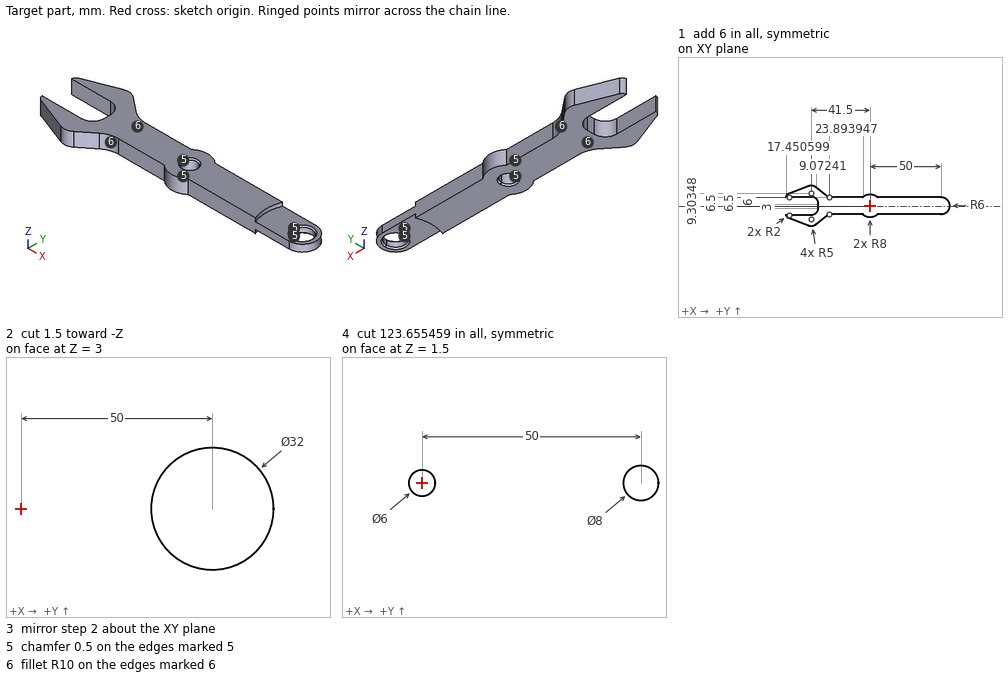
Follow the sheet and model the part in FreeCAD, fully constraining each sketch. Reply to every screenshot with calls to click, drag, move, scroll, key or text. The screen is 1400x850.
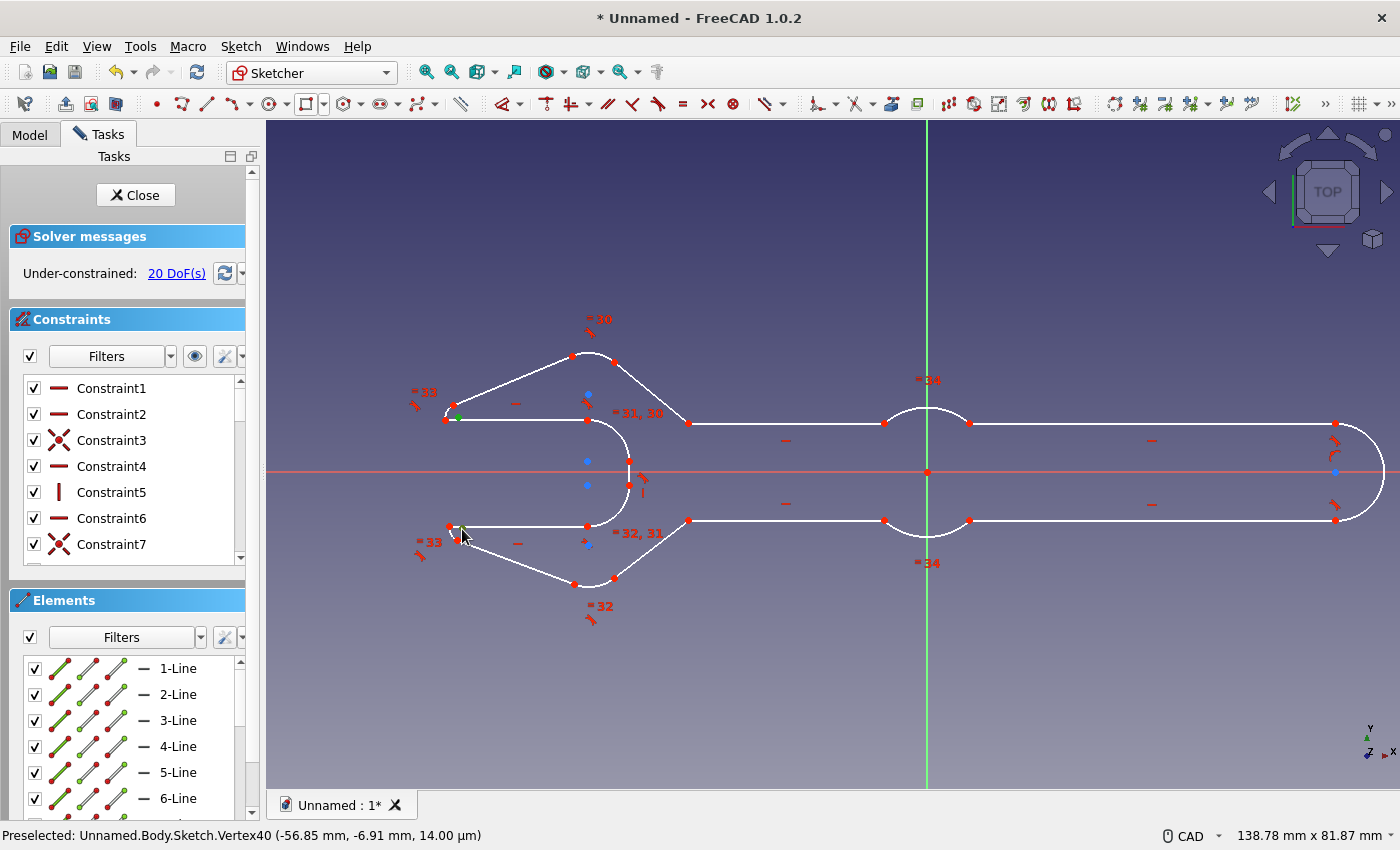
click(361, 472)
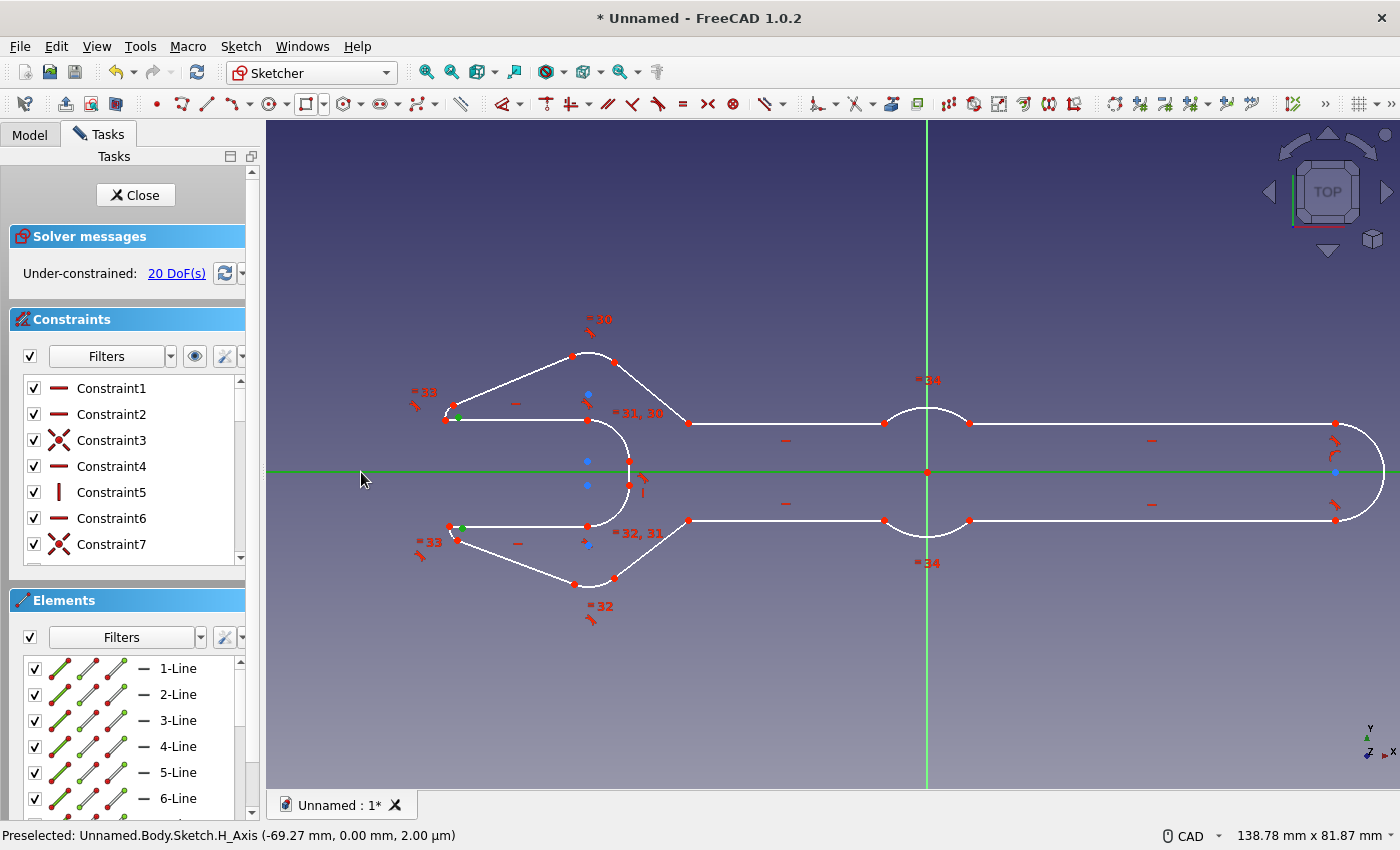
click(708, 104)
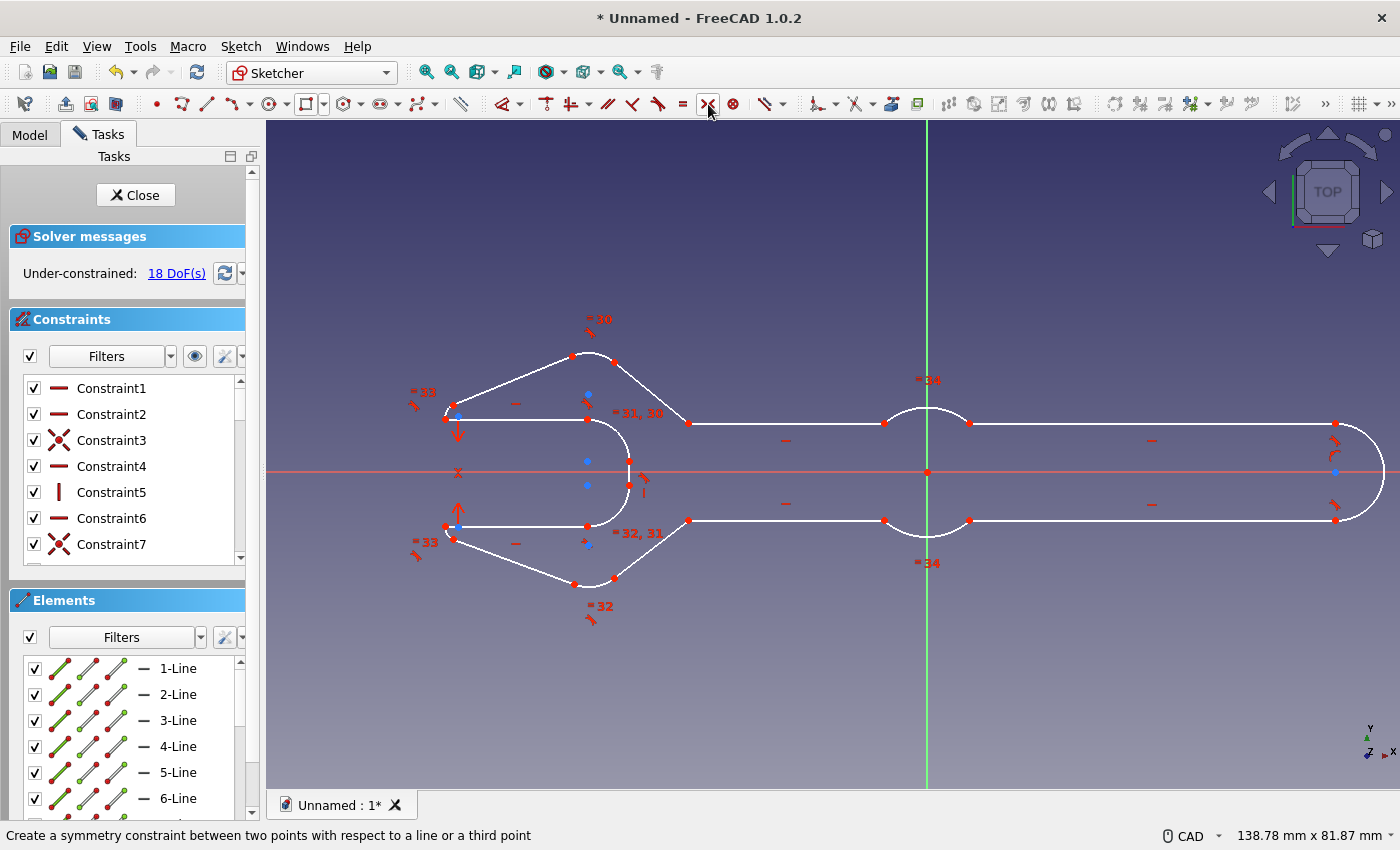
click(588, 394)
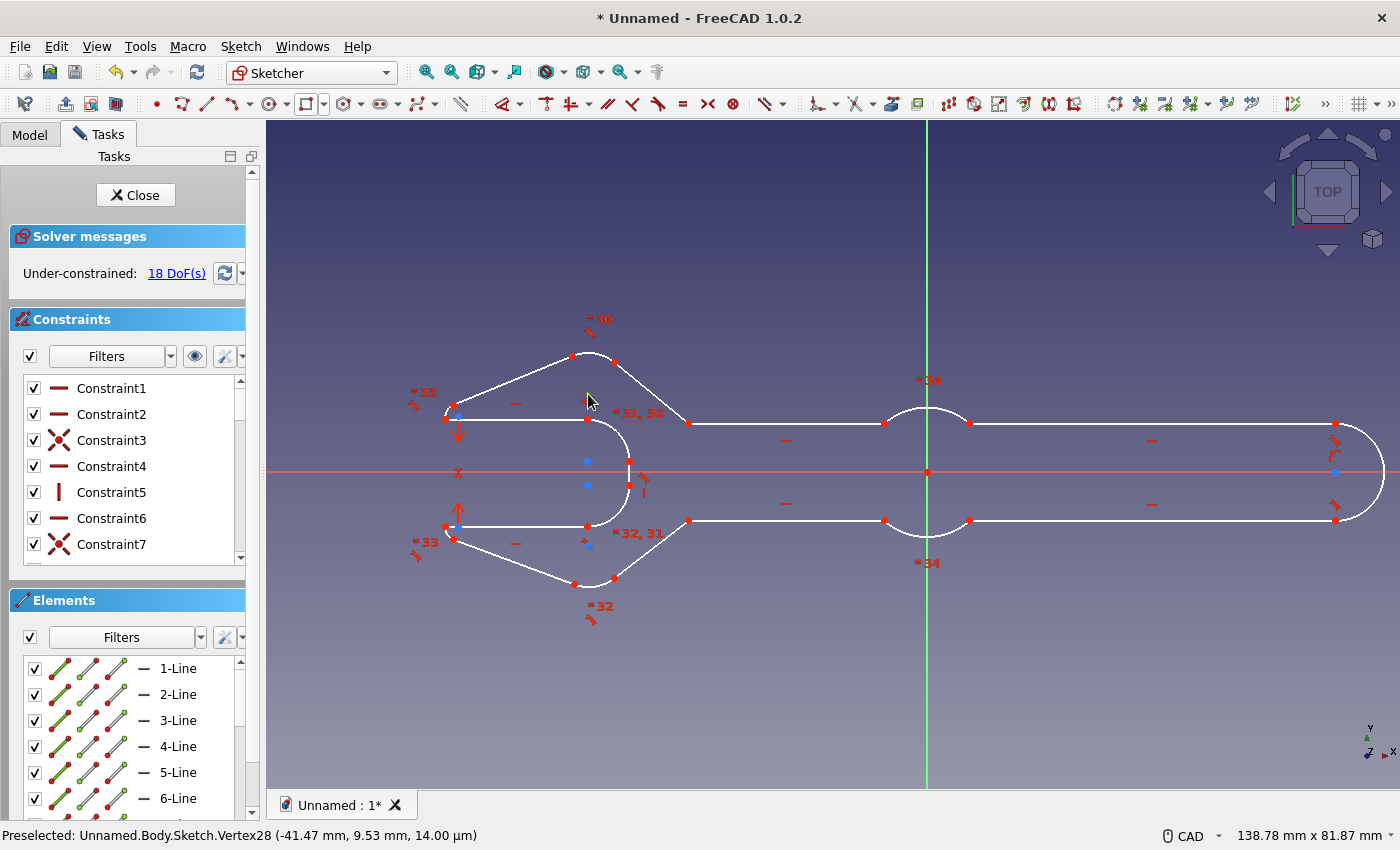
click(589, 546)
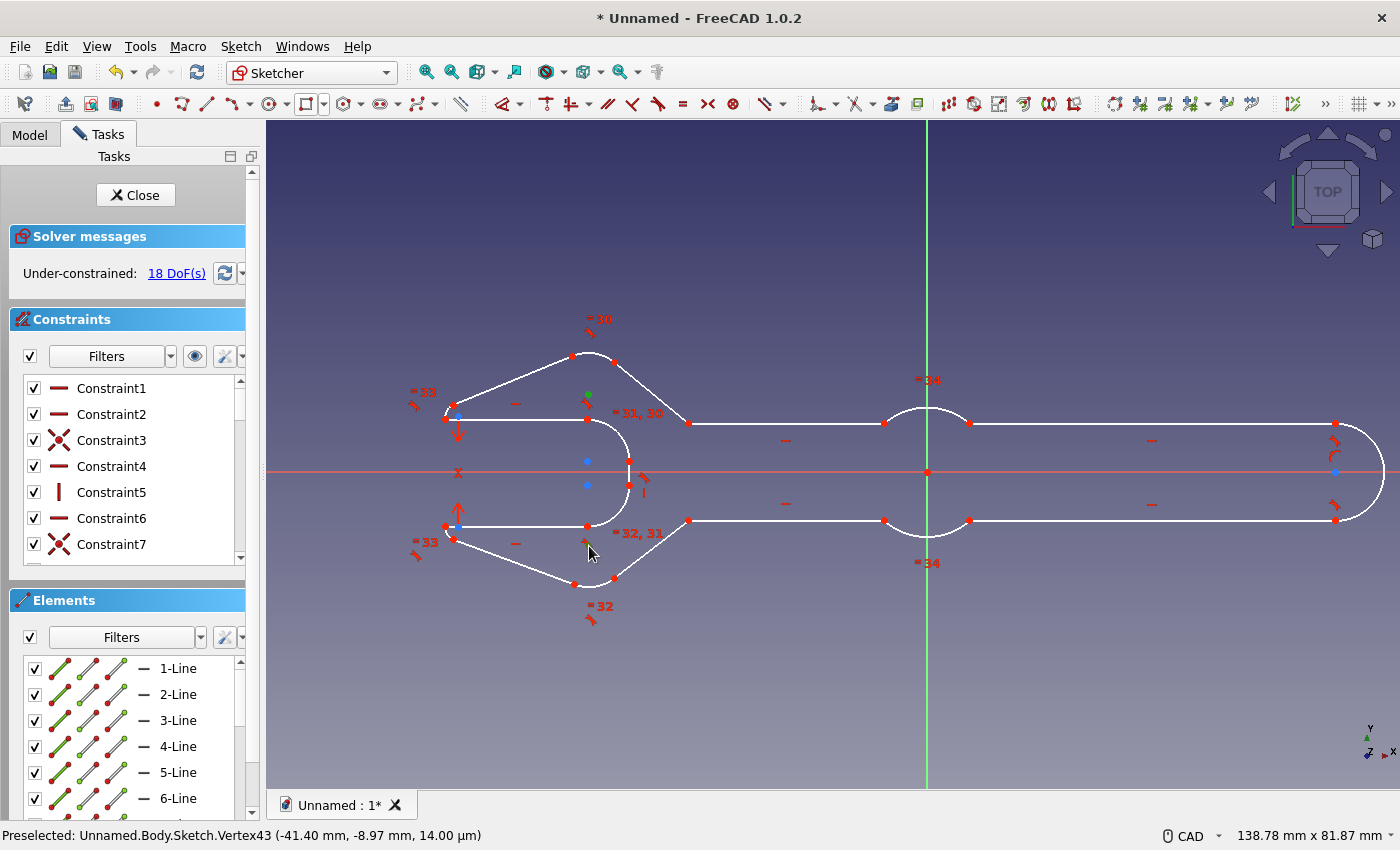
click(361, 472)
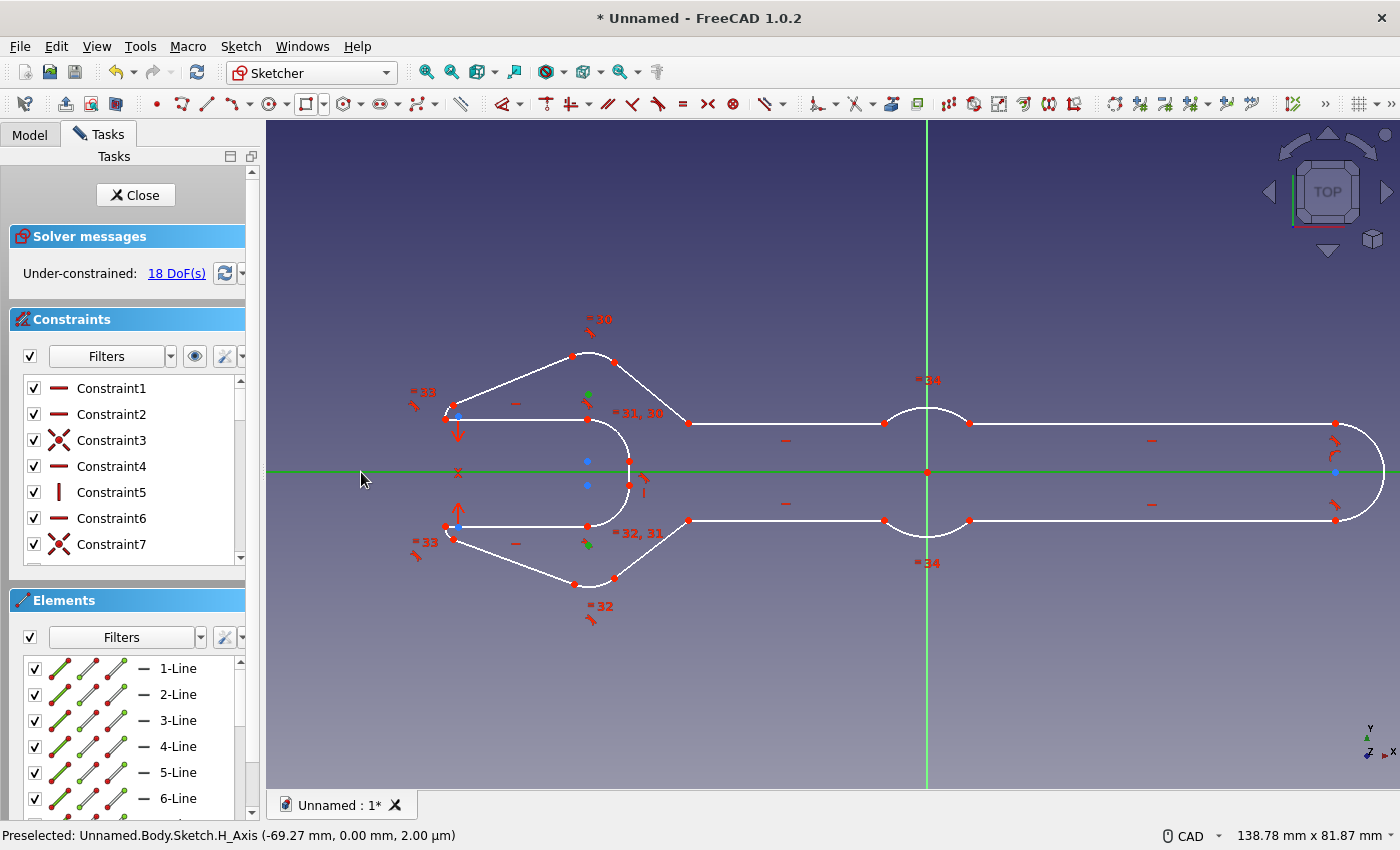
click(708, 104)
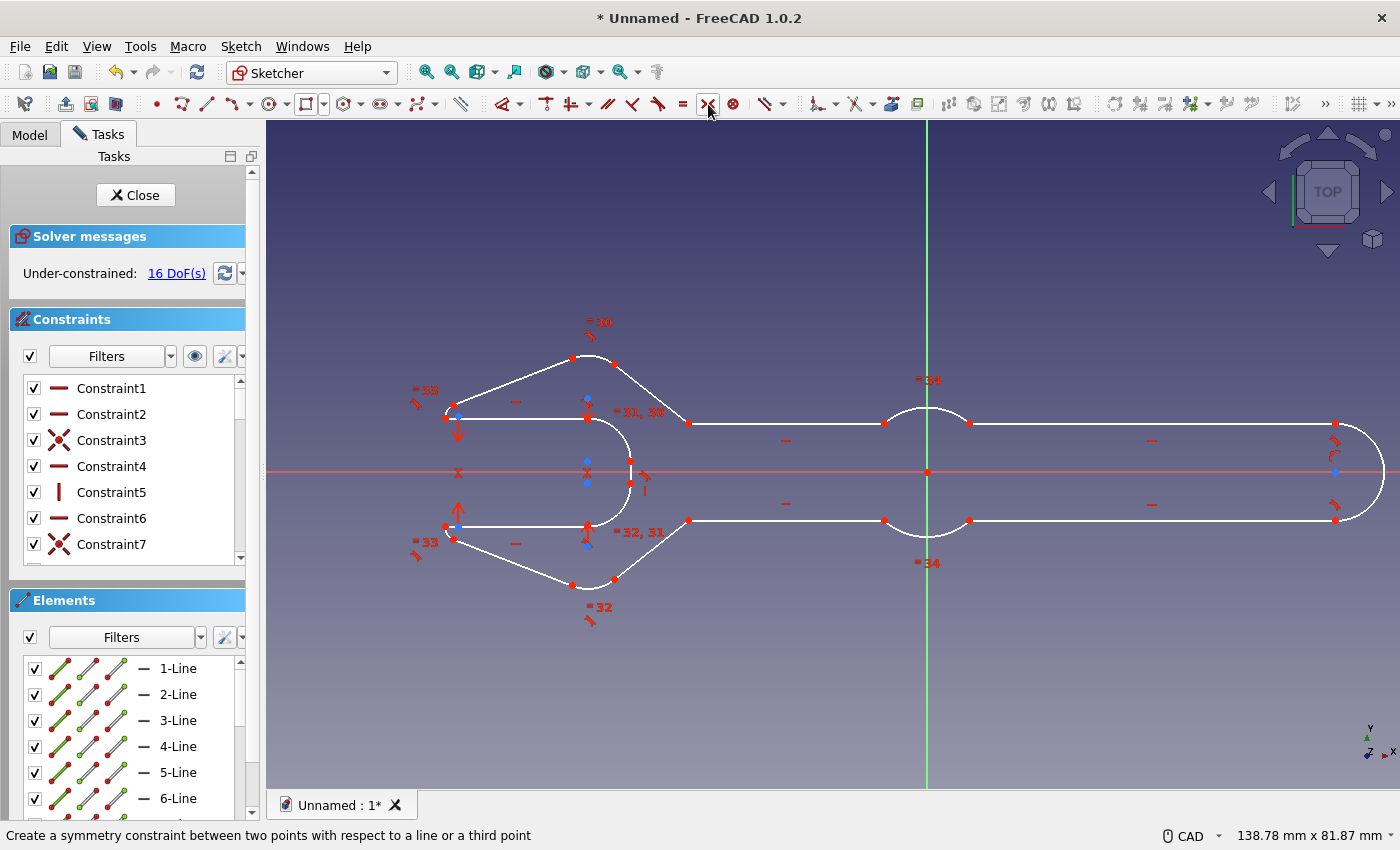
click(689, 424)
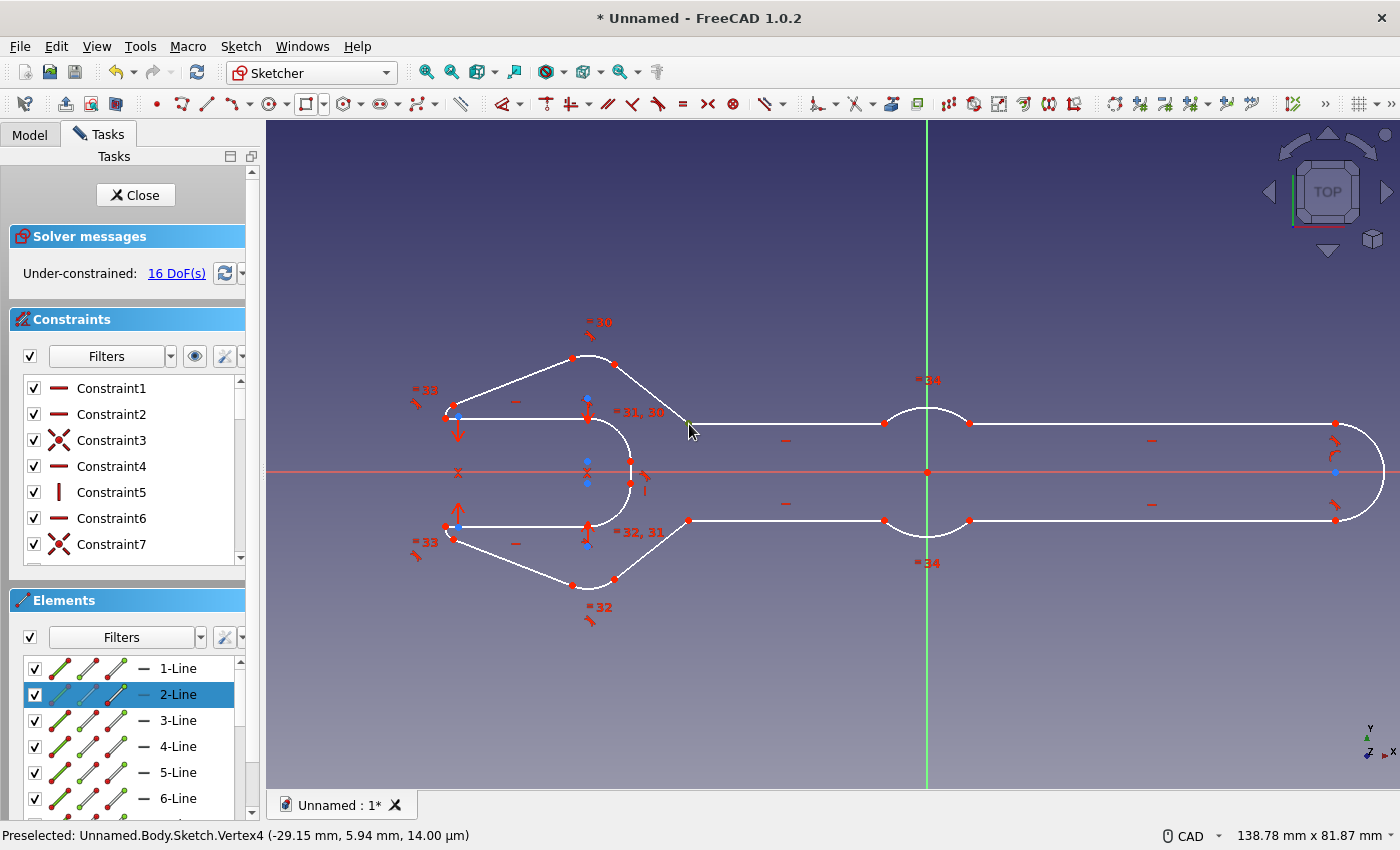
click(689, 521)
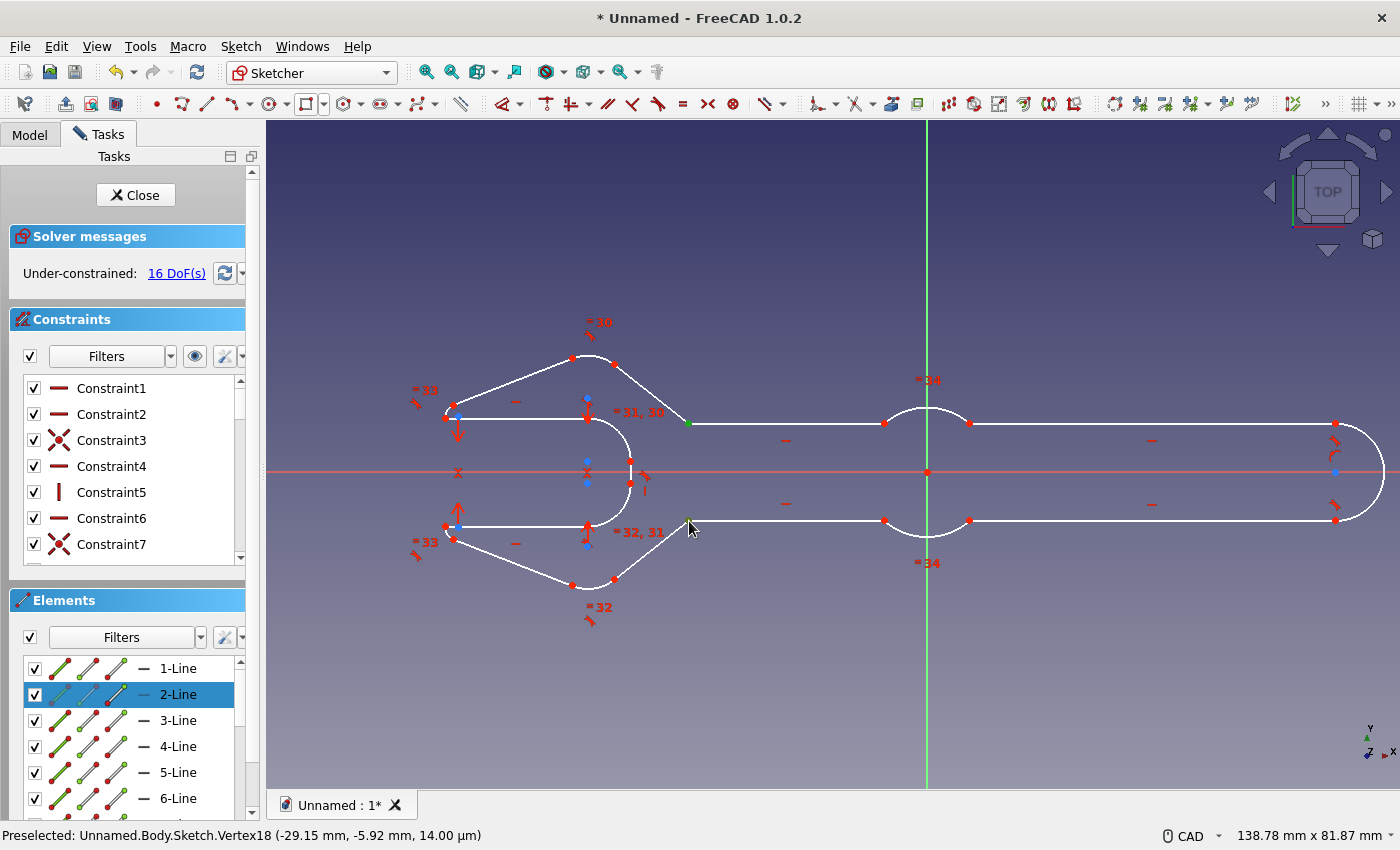
click(361, 472)